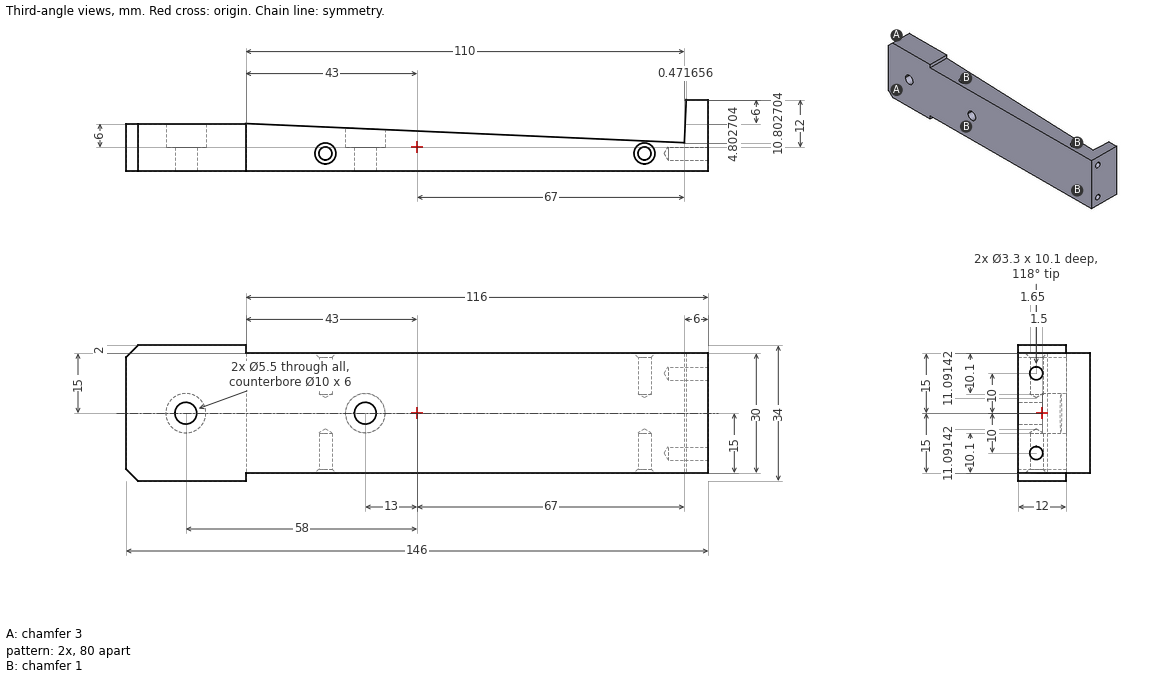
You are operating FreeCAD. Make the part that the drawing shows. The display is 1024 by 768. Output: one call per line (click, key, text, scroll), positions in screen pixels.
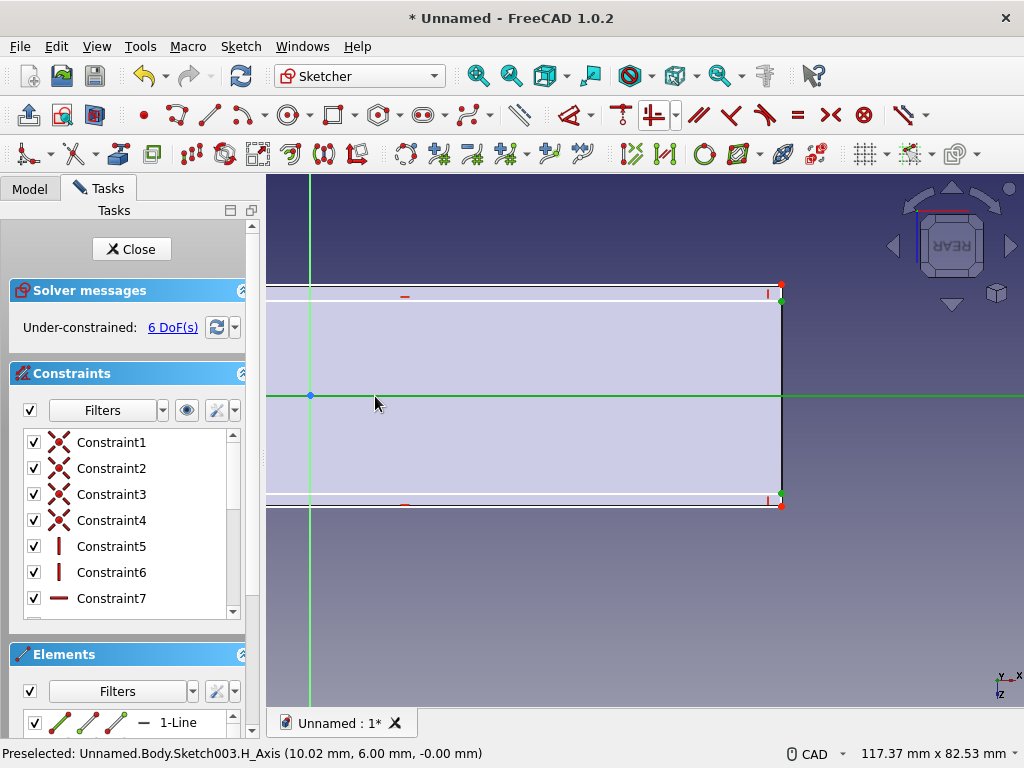
click(831, 116)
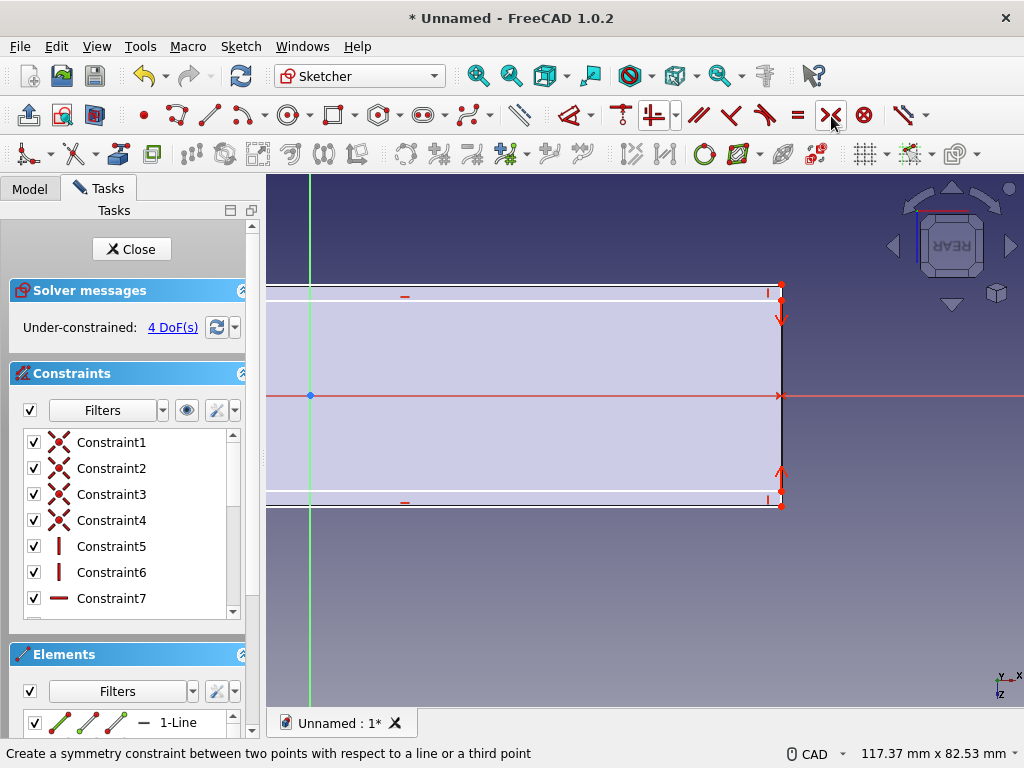
key(d)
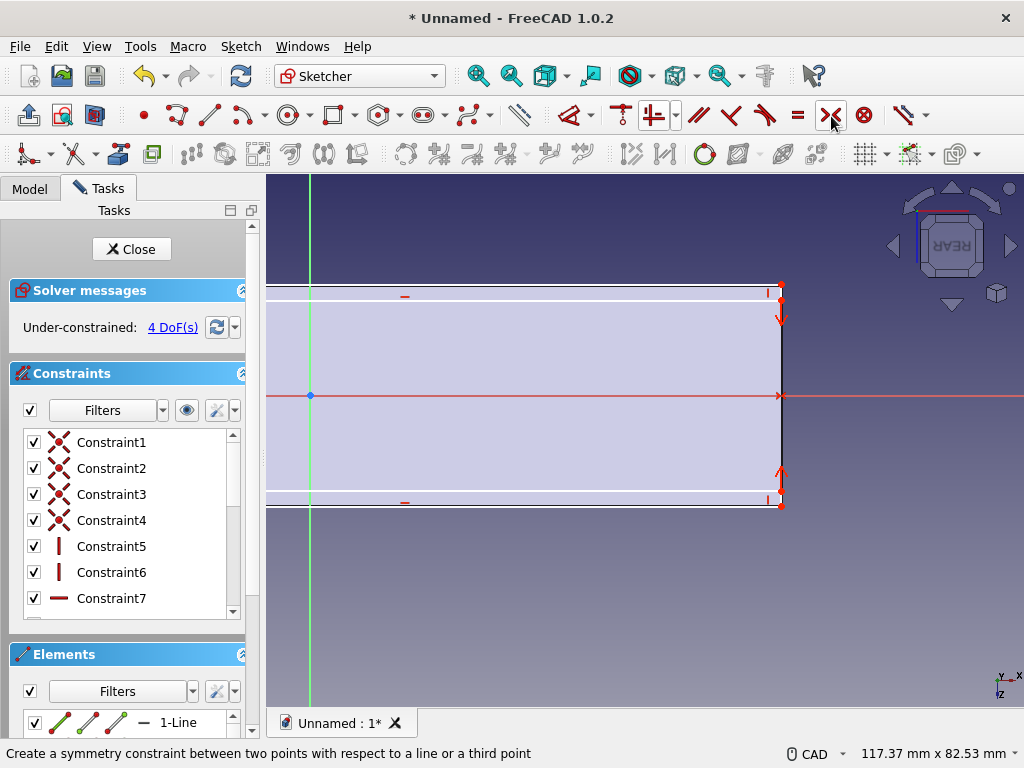
scroll(783, 495, down, 3)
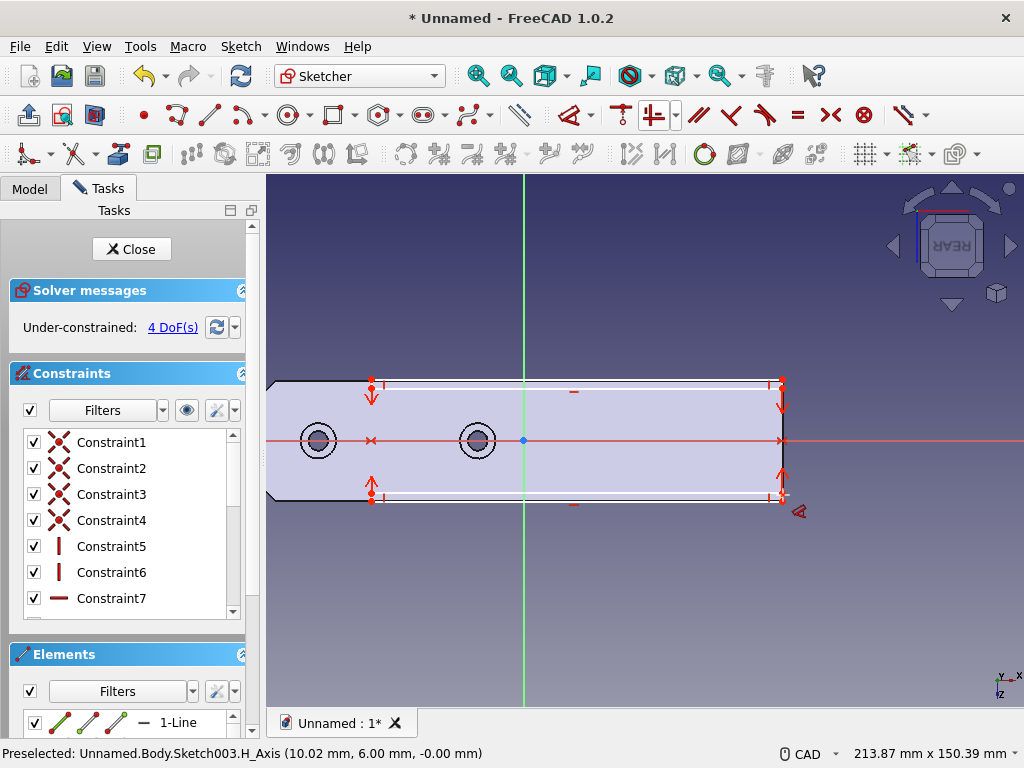
scroll(372, 497, up, 9)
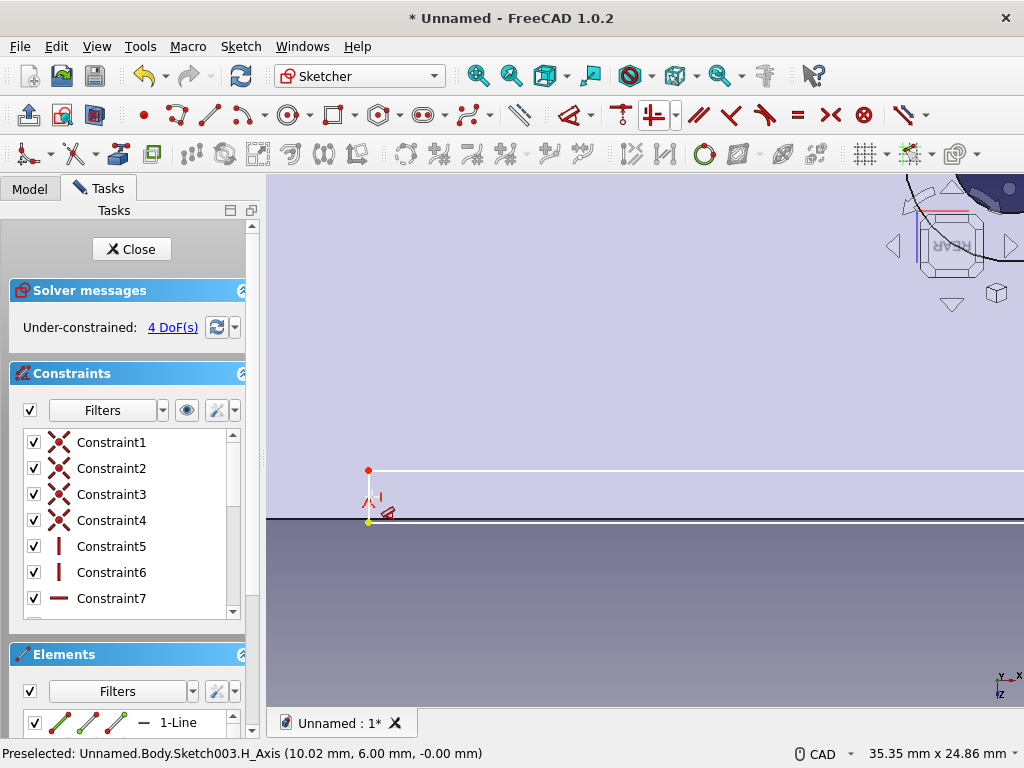
click(369, 497)
click(335, 497)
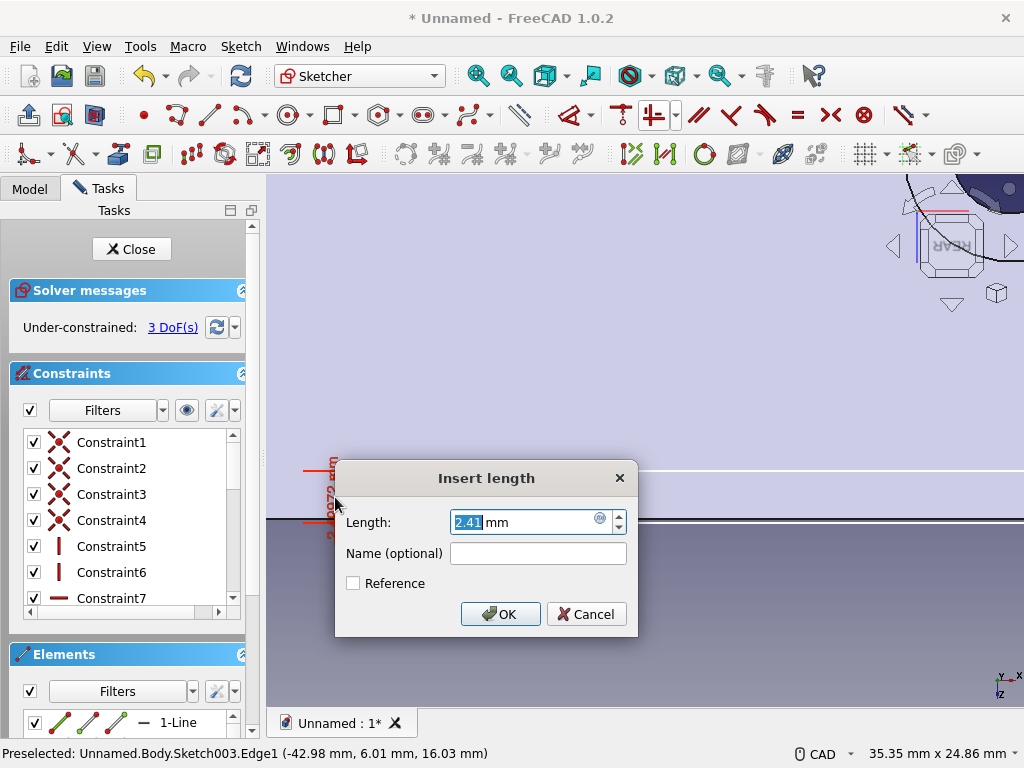
text(2)
key(Return)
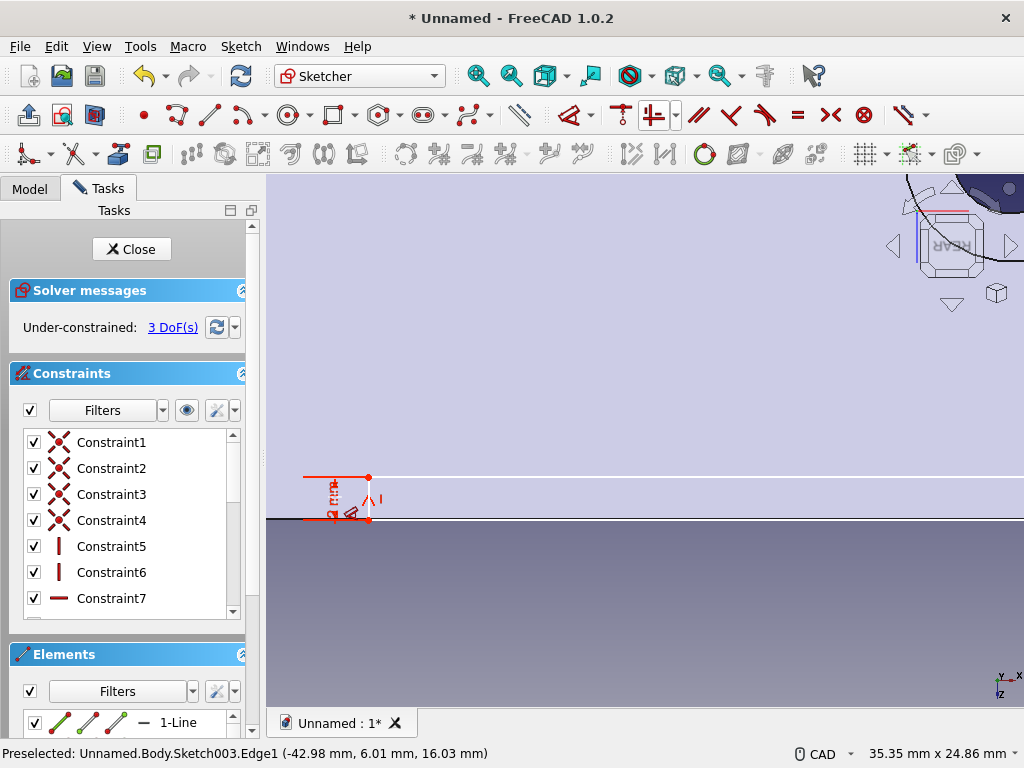
scroll(372, 497, down, 9)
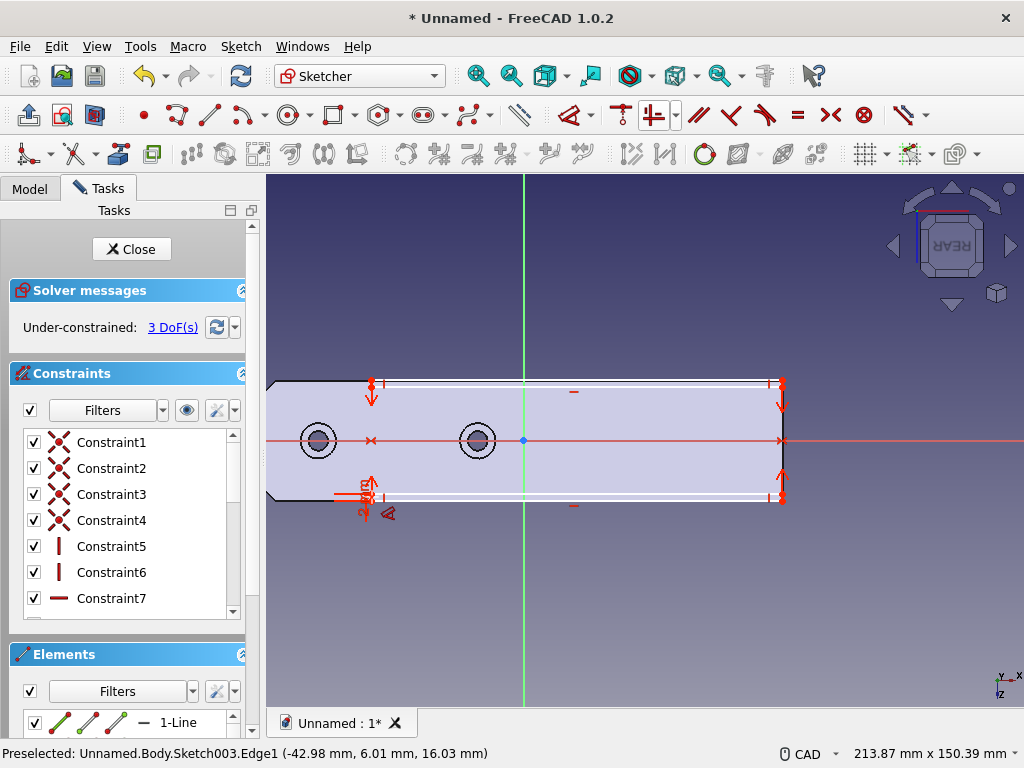
scroll(495, 501, up, 4)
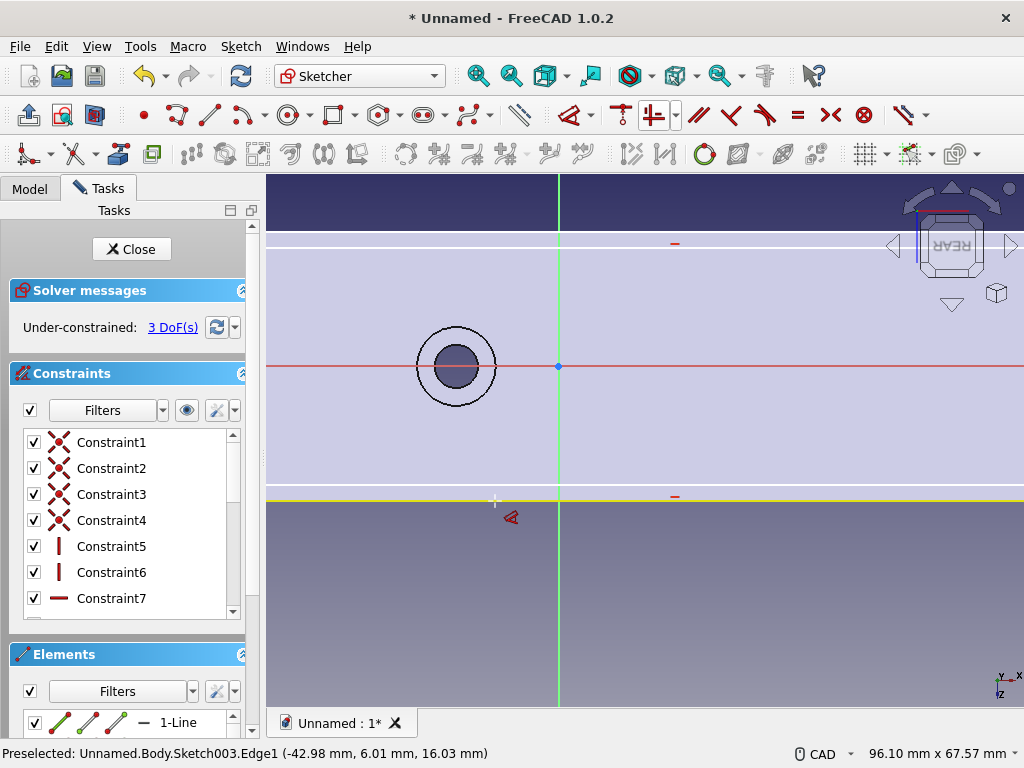
click(494, 501)
click(576, 535)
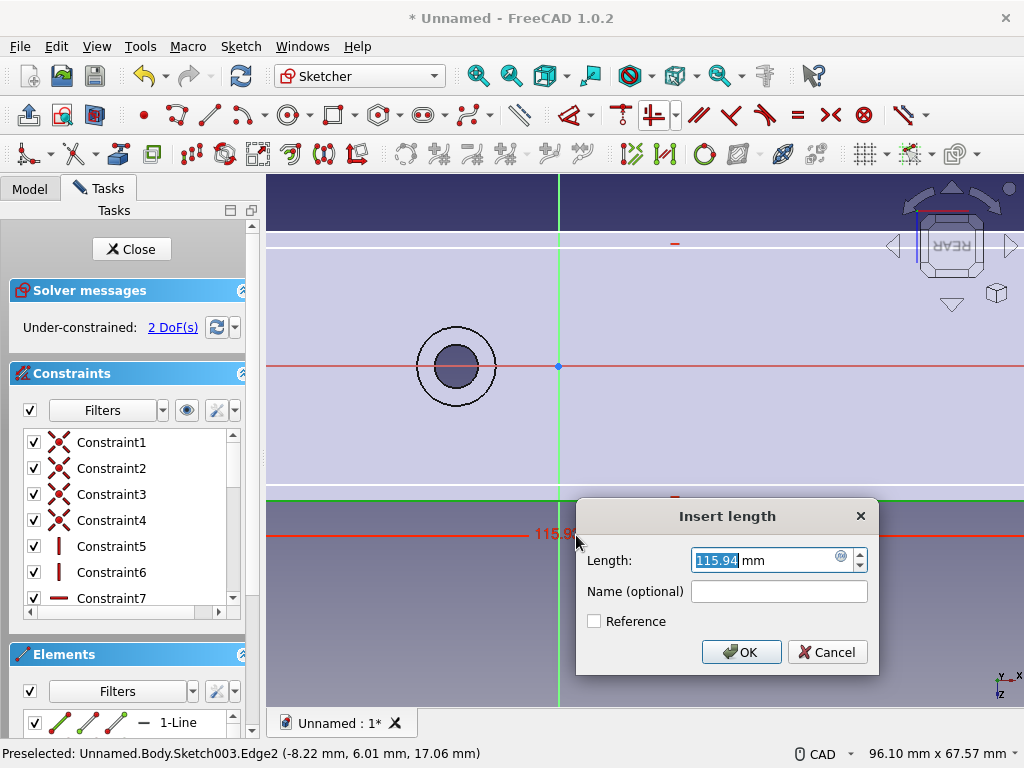
text(116)
key(Return)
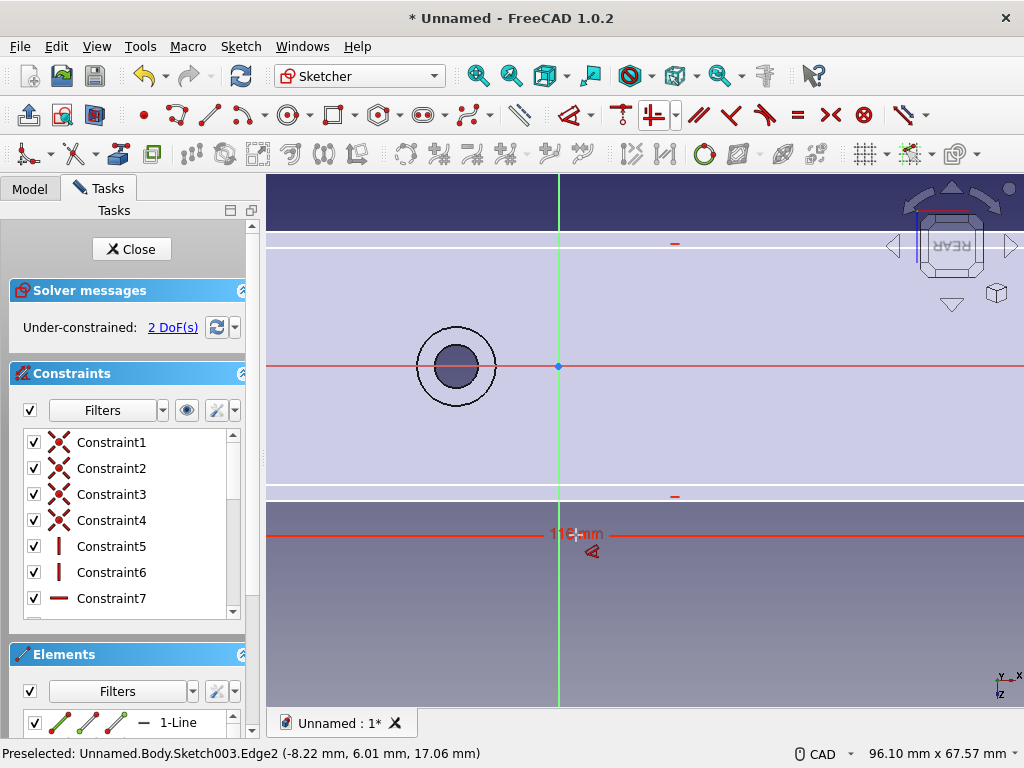
scroll(494, 501, down, 4)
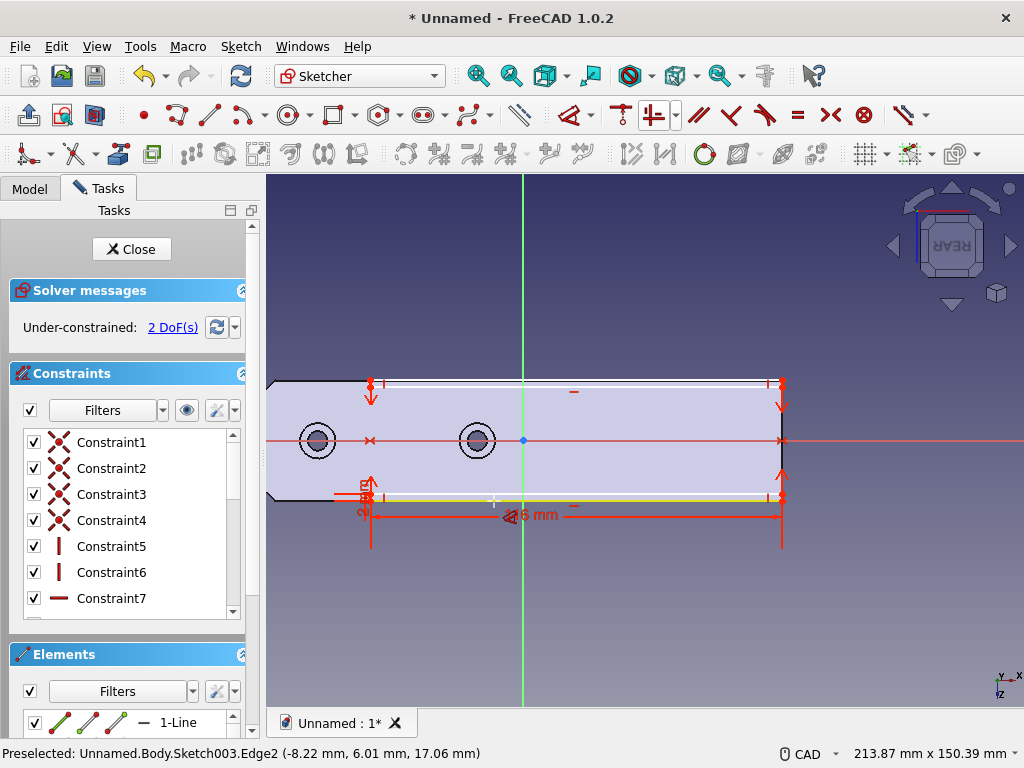
scroll(371, 494, up, 3)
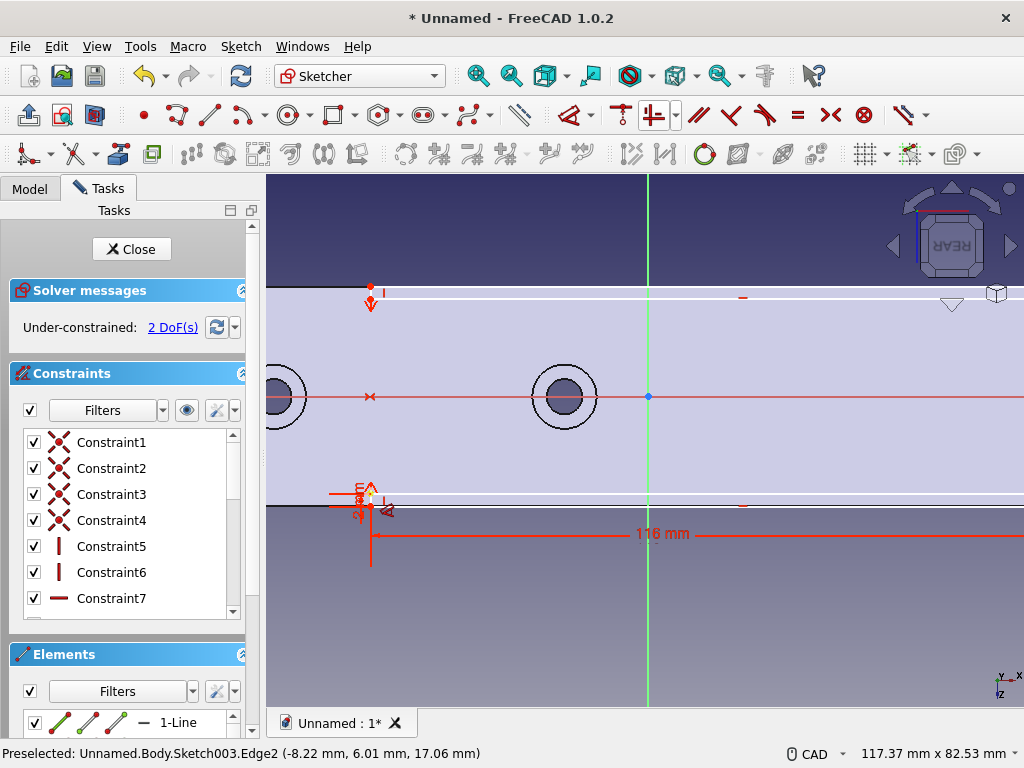
click(371, 494)
click(510, 528)